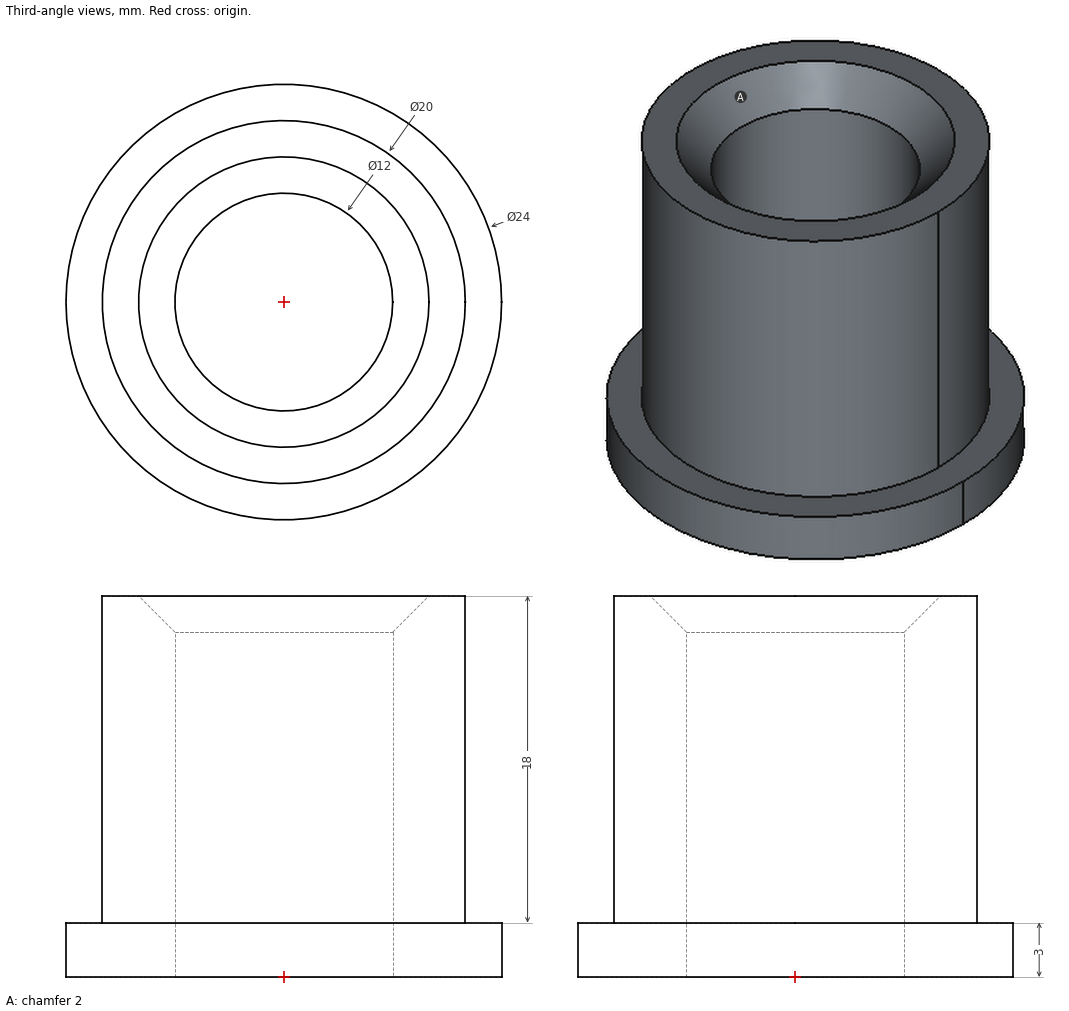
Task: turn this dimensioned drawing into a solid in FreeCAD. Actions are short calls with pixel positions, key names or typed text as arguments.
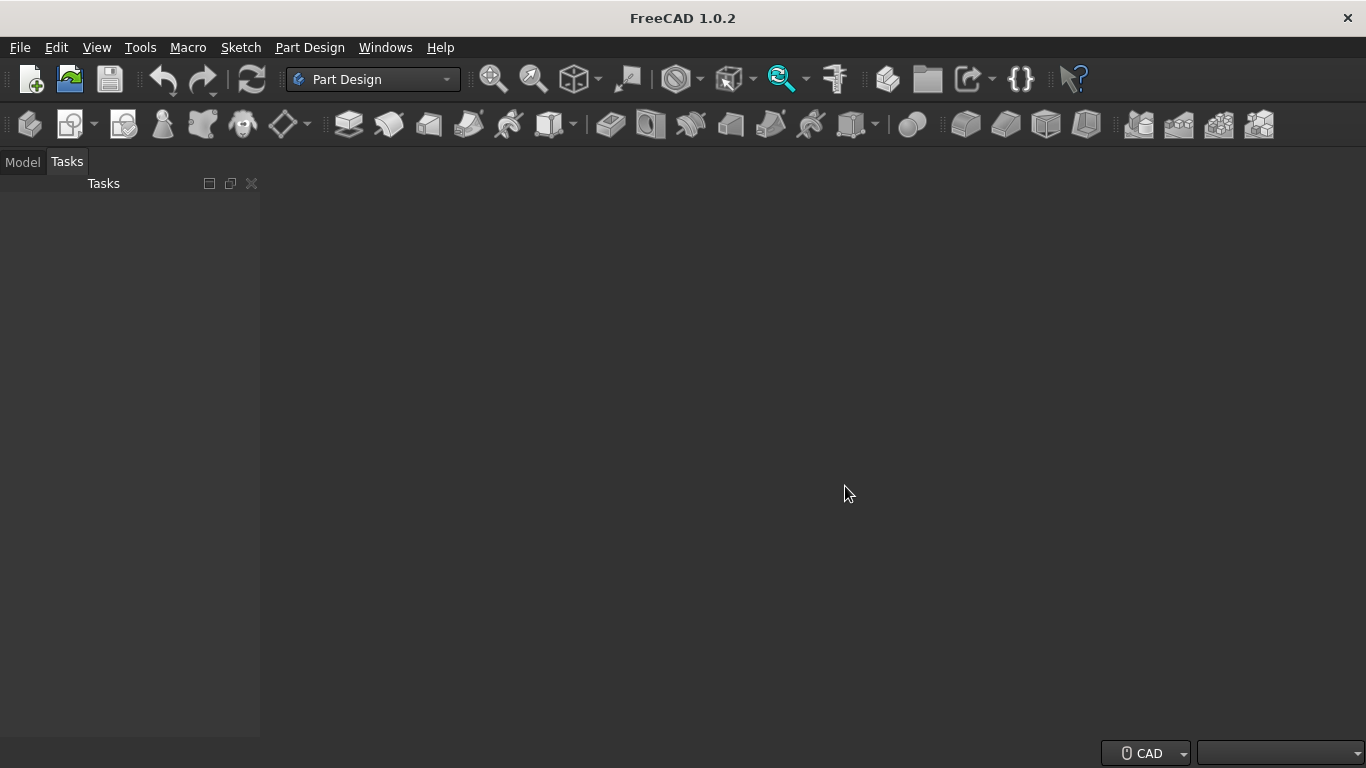
click(30, 80)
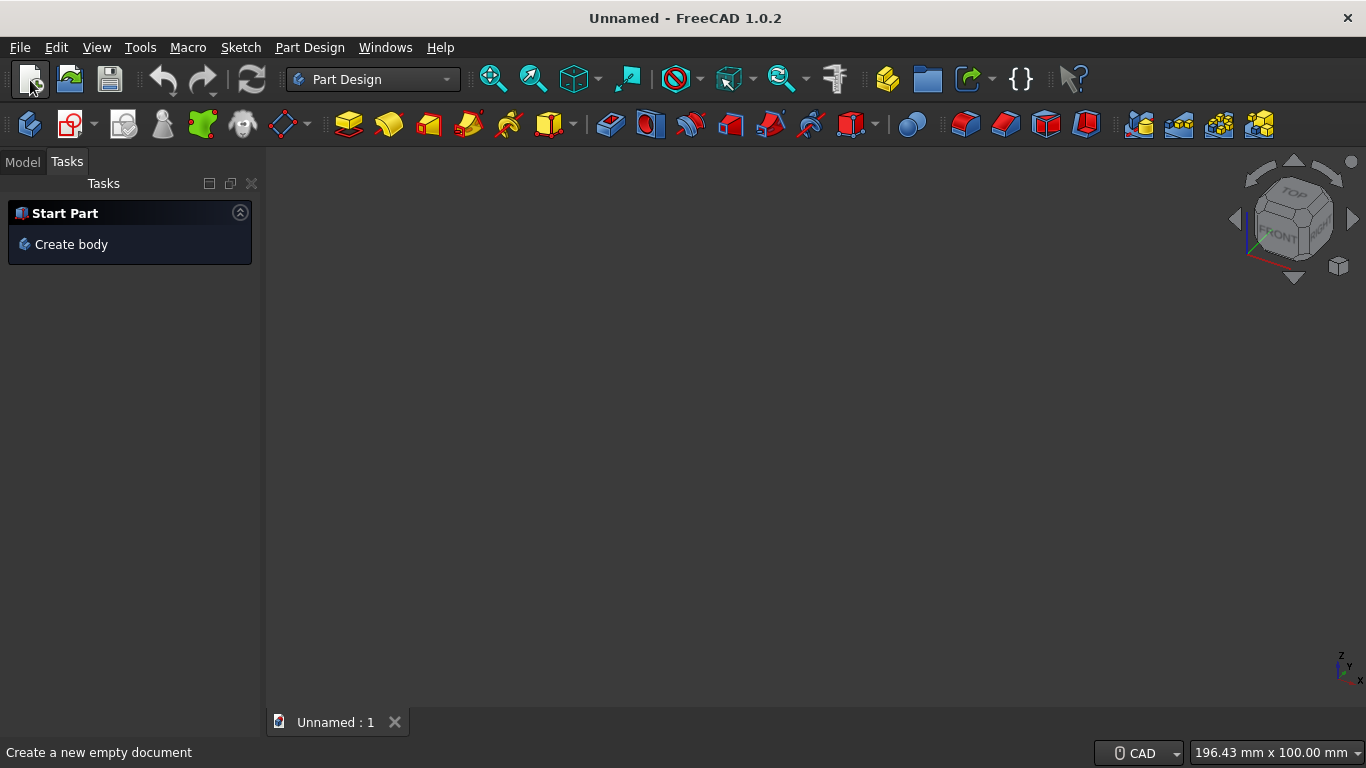
click(70, 124)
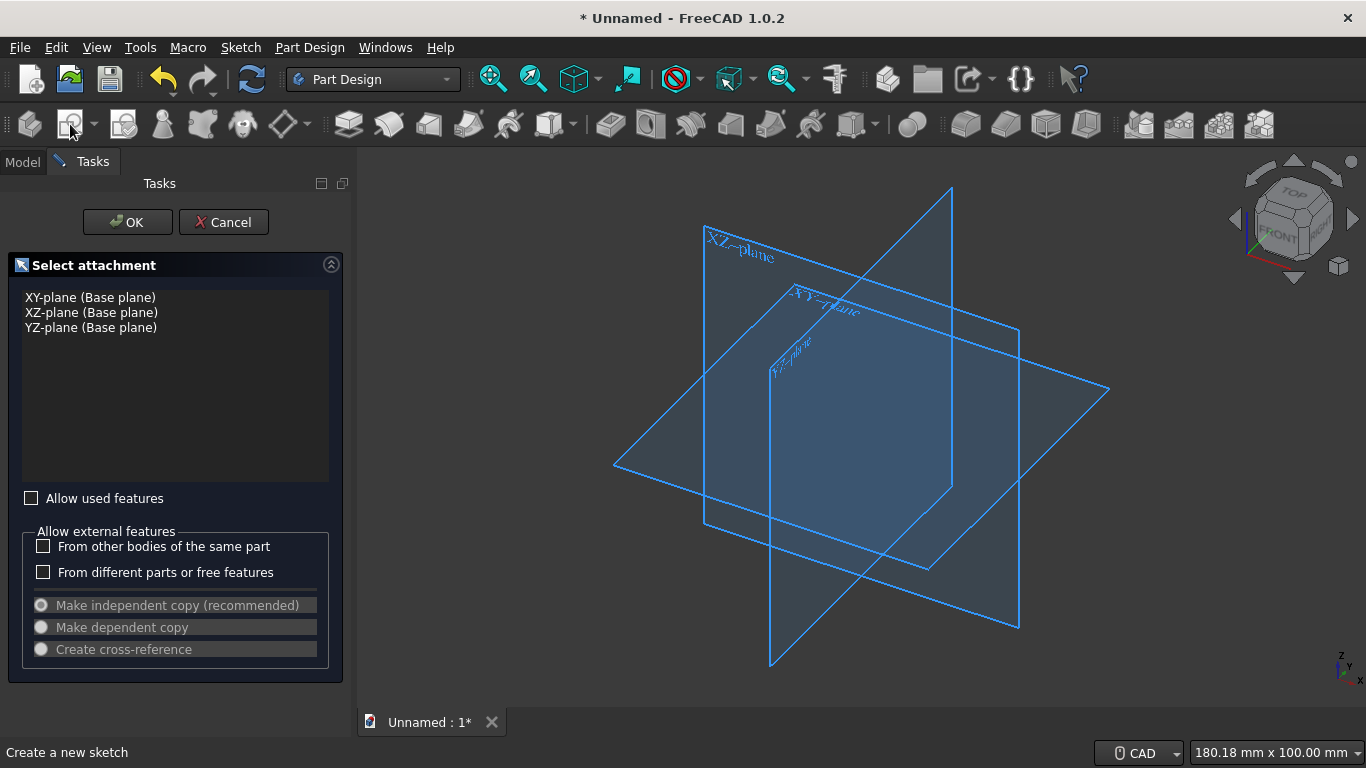
click(82, 298)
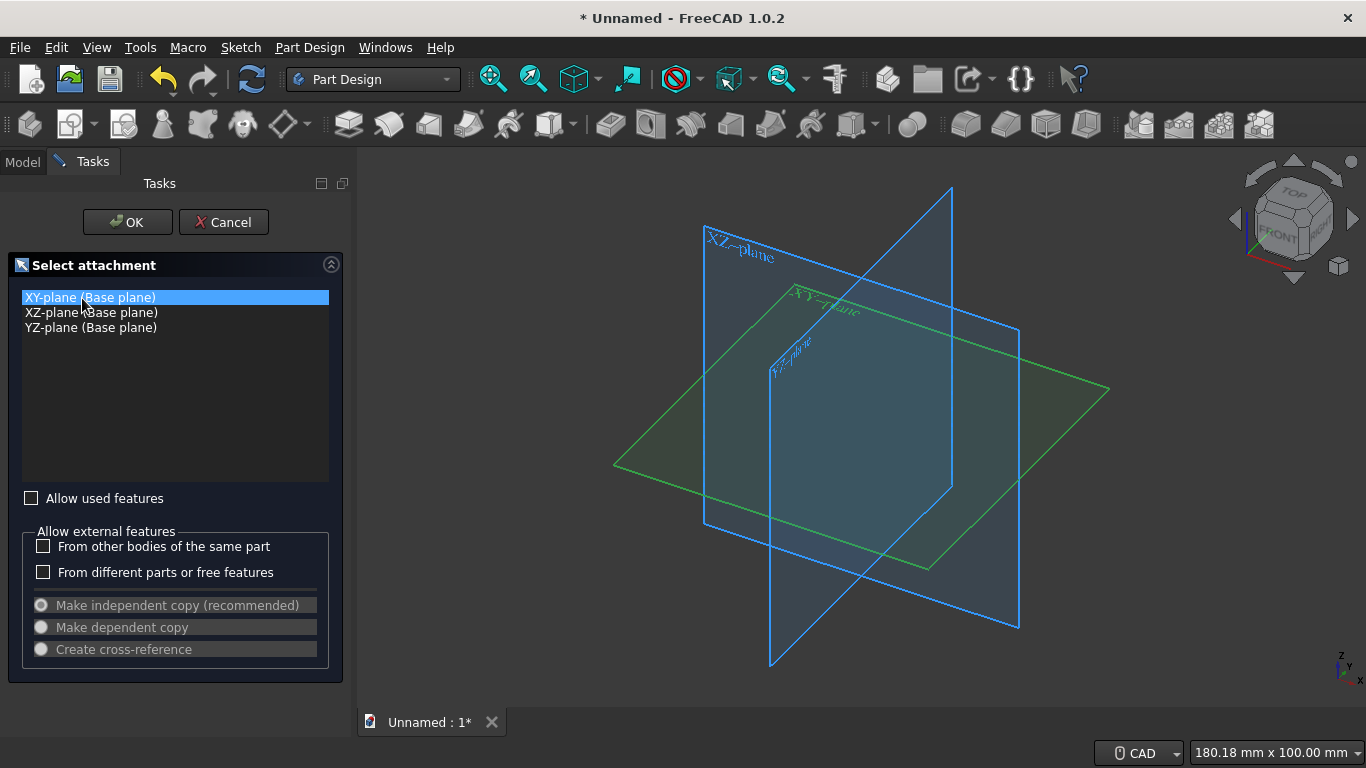
click(128, 222)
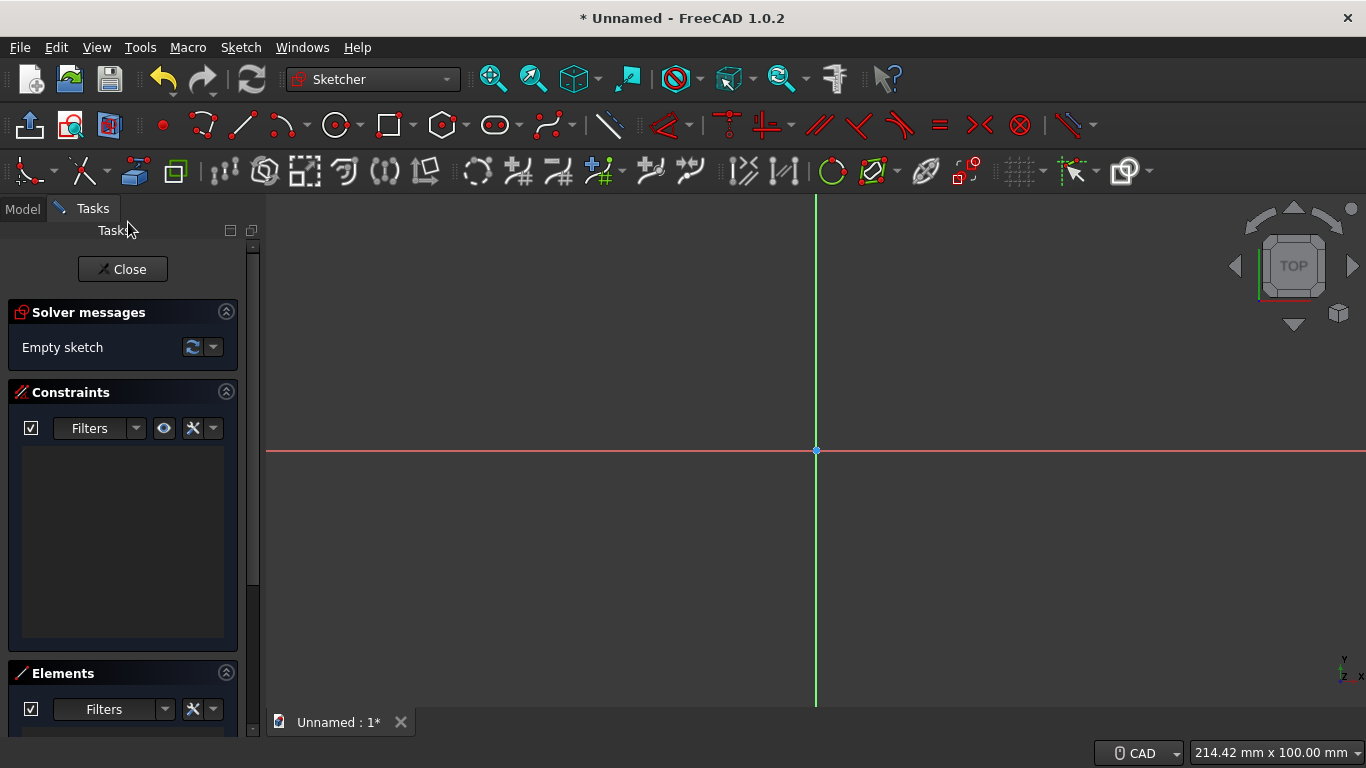
scroll(856, 450, up, 5)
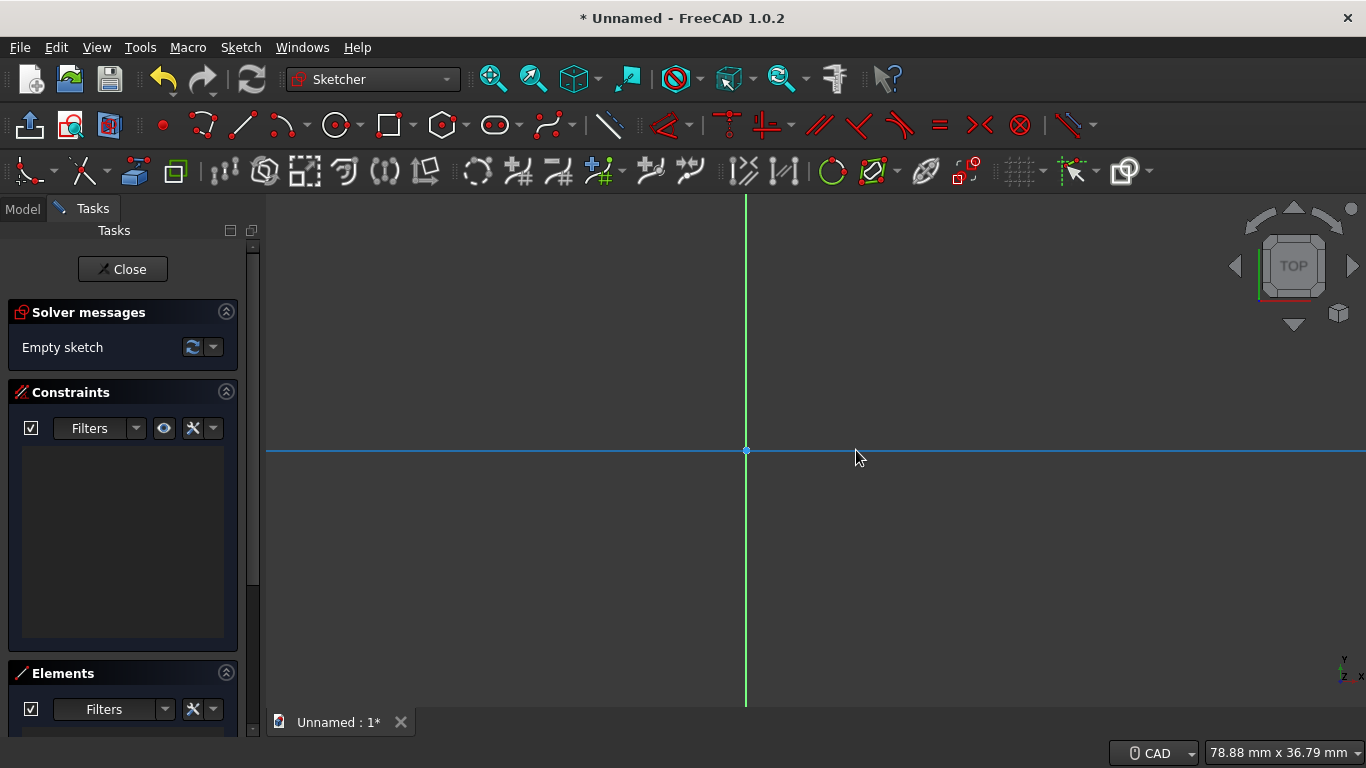
click(336, 126)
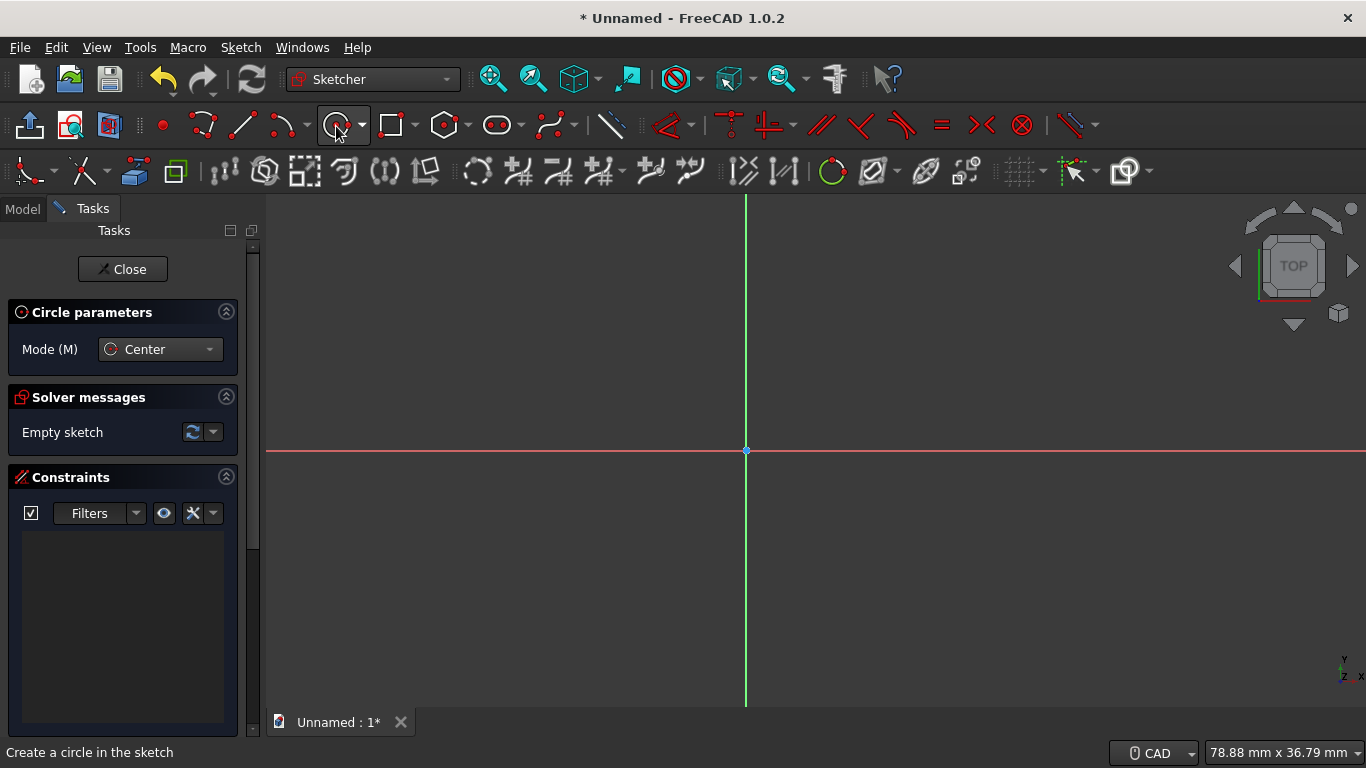
click(746, 450)
move(865, 332)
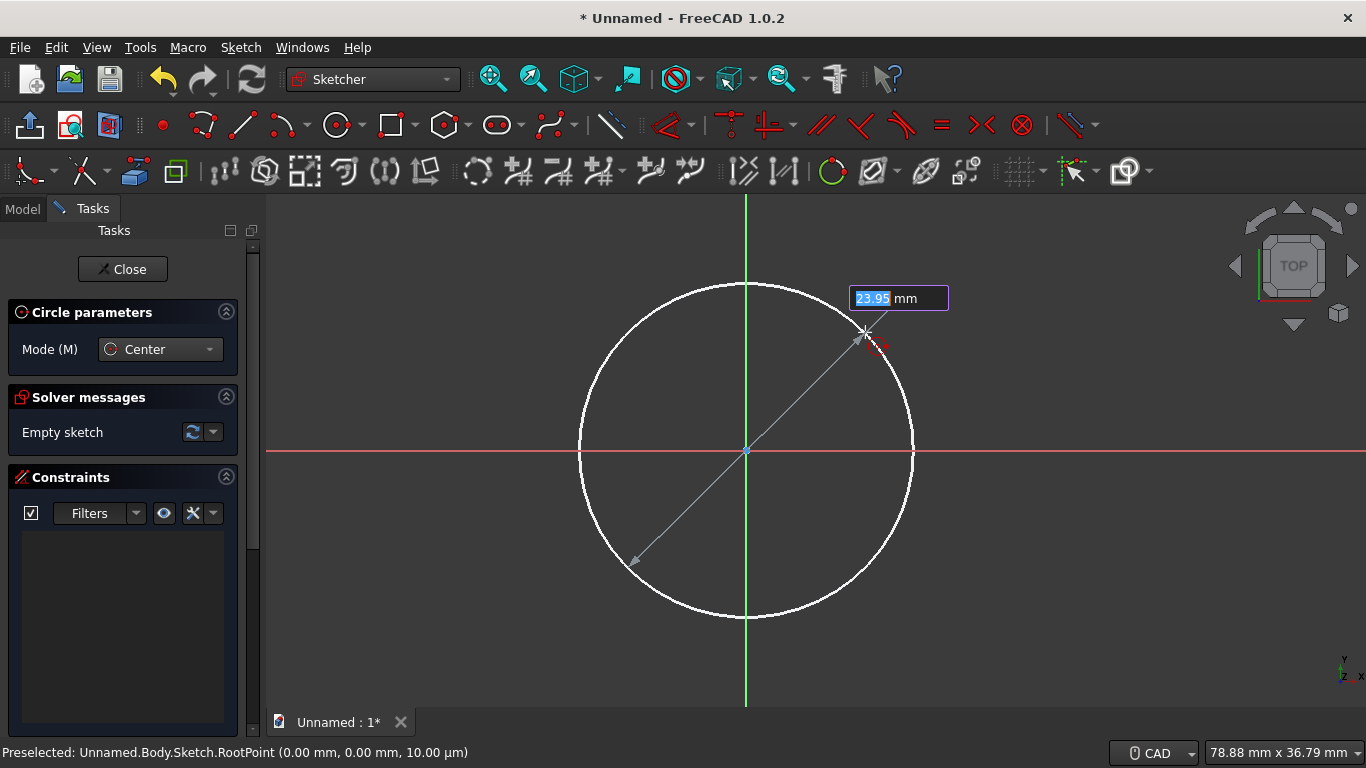
text(24)
key(Return)
key(Escape)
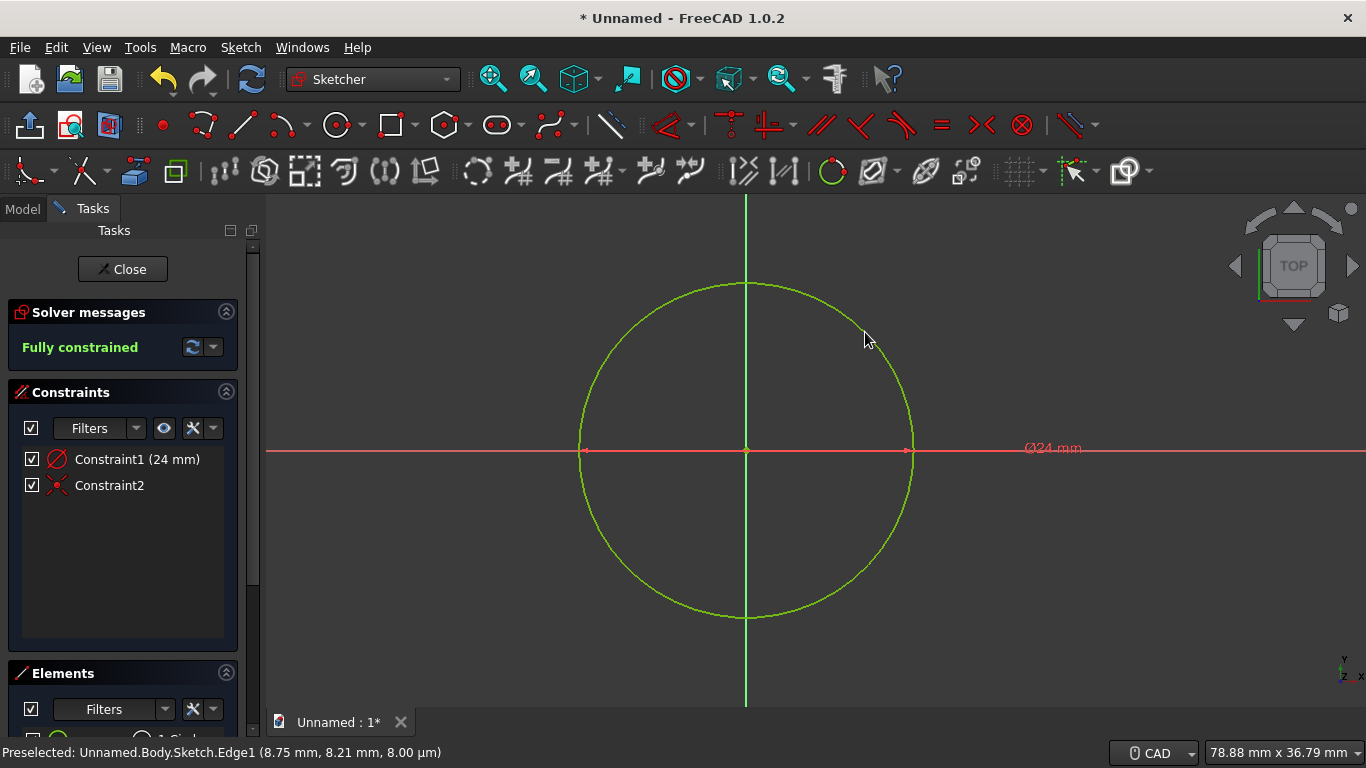
click(123, 269)